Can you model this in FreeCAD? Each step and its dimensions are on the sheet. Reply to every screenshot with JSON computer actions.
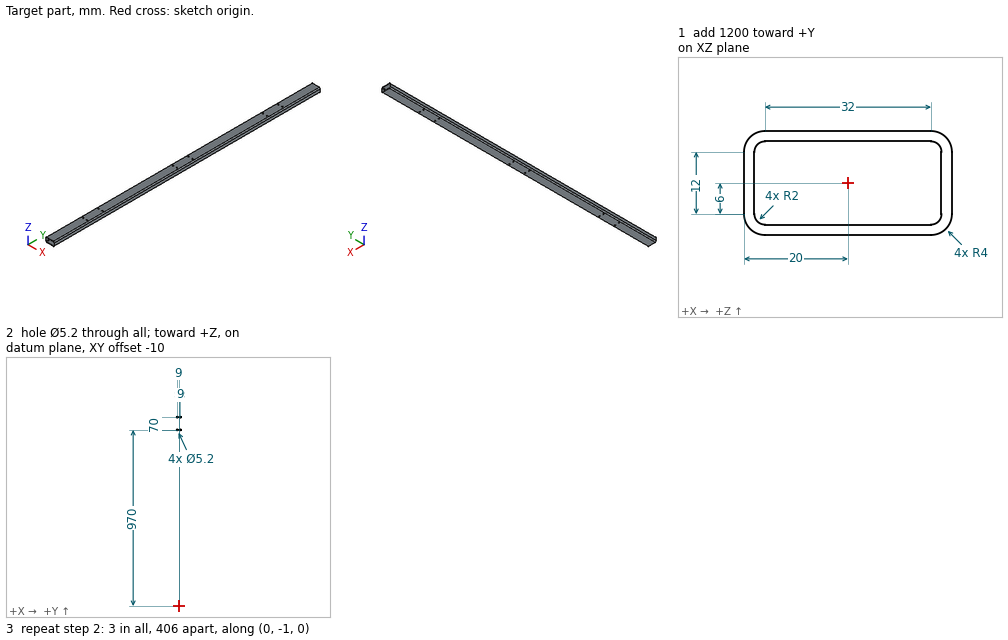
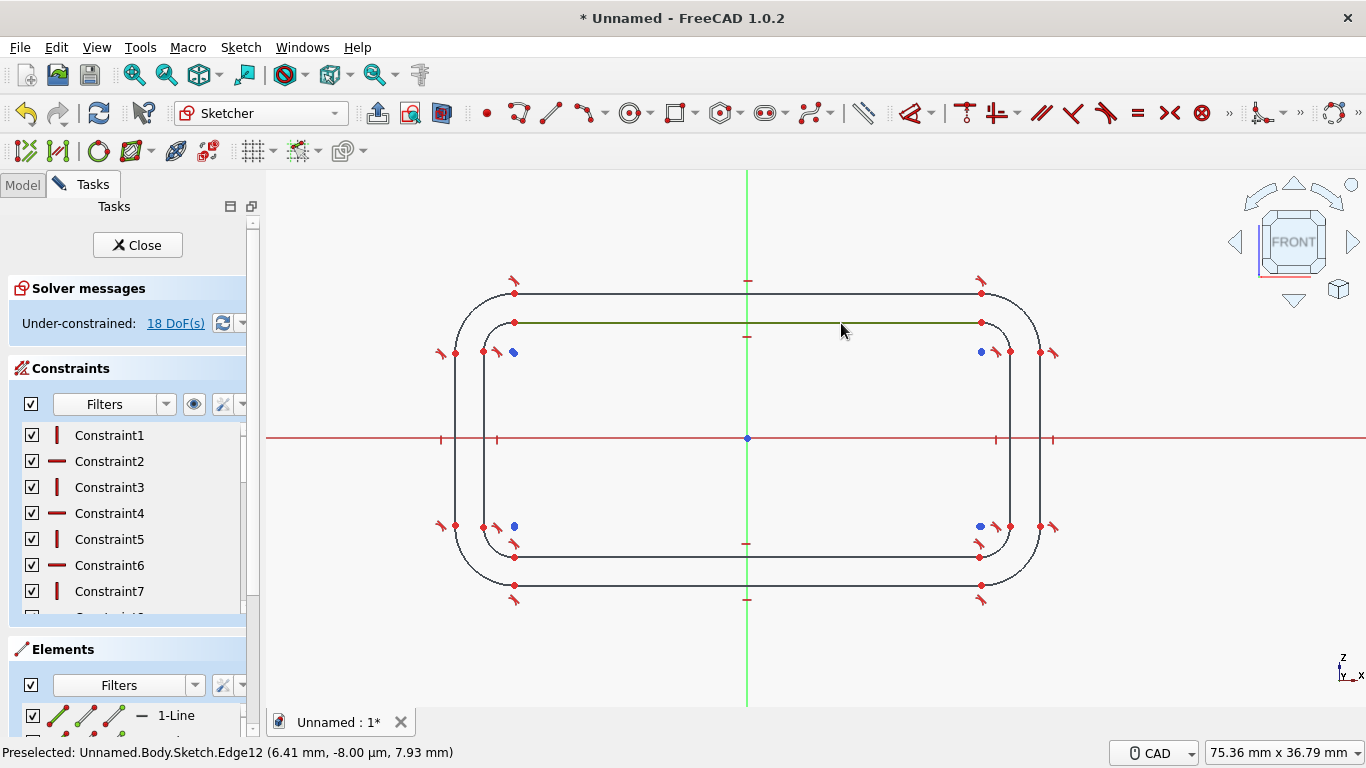
{"action": "left_click", "coordinate": [1007, 338]}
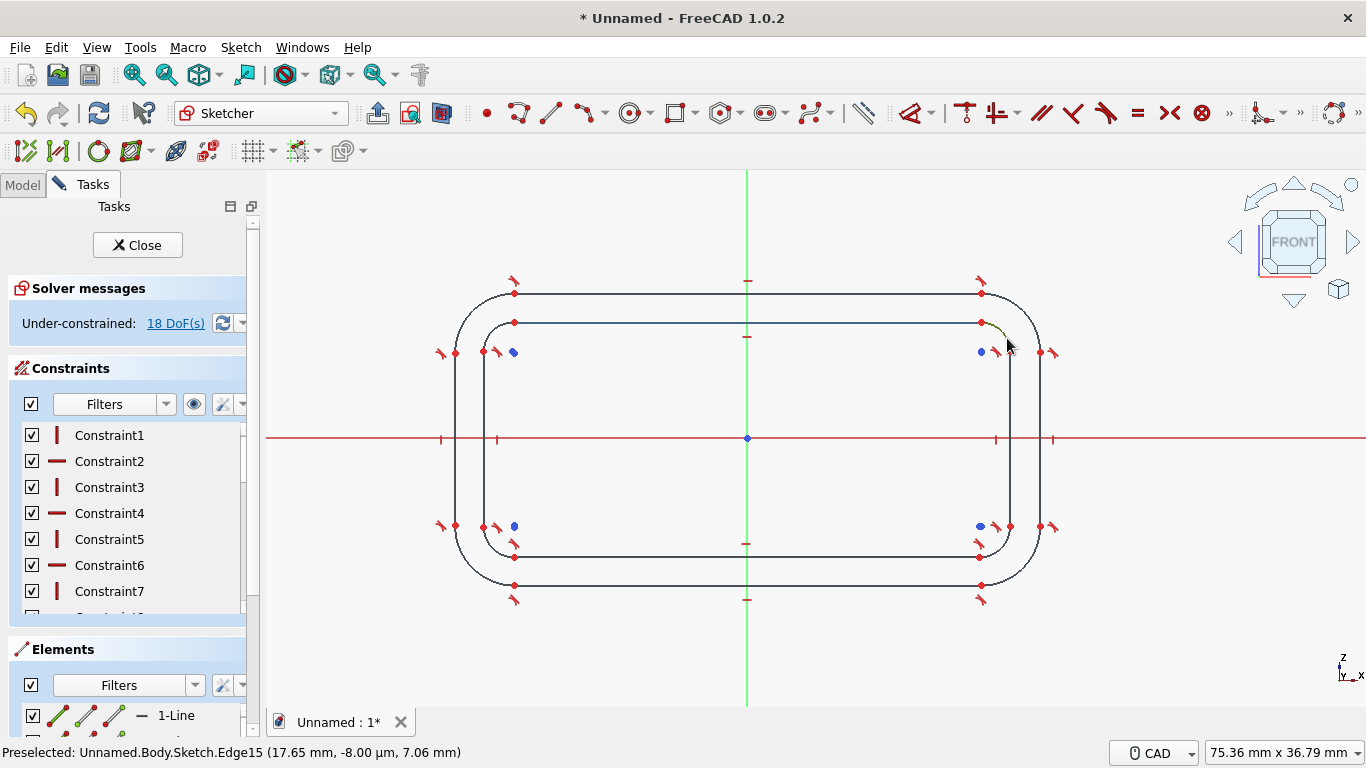
{"action": "left_click", "coordinate": [1106, 114]}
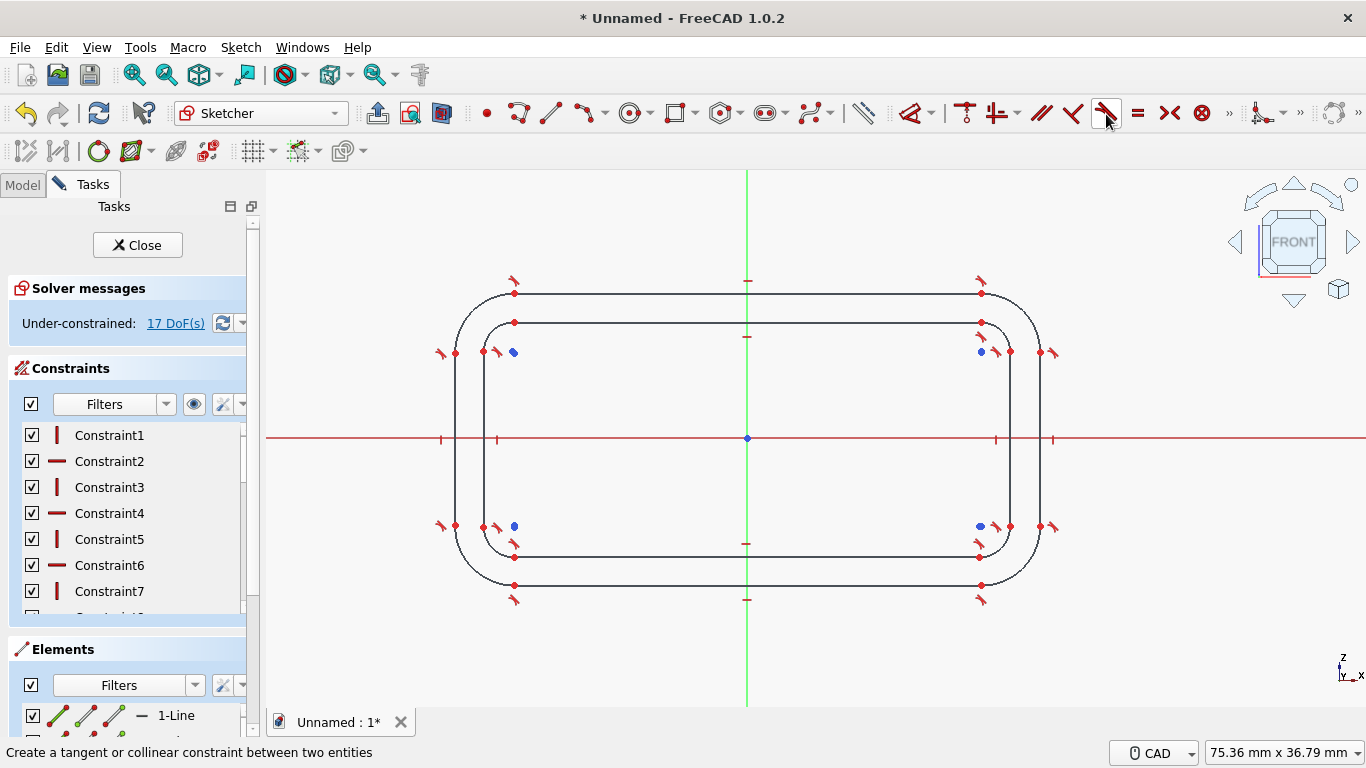
{"action": "left_click", "coordinate": [841, 323]}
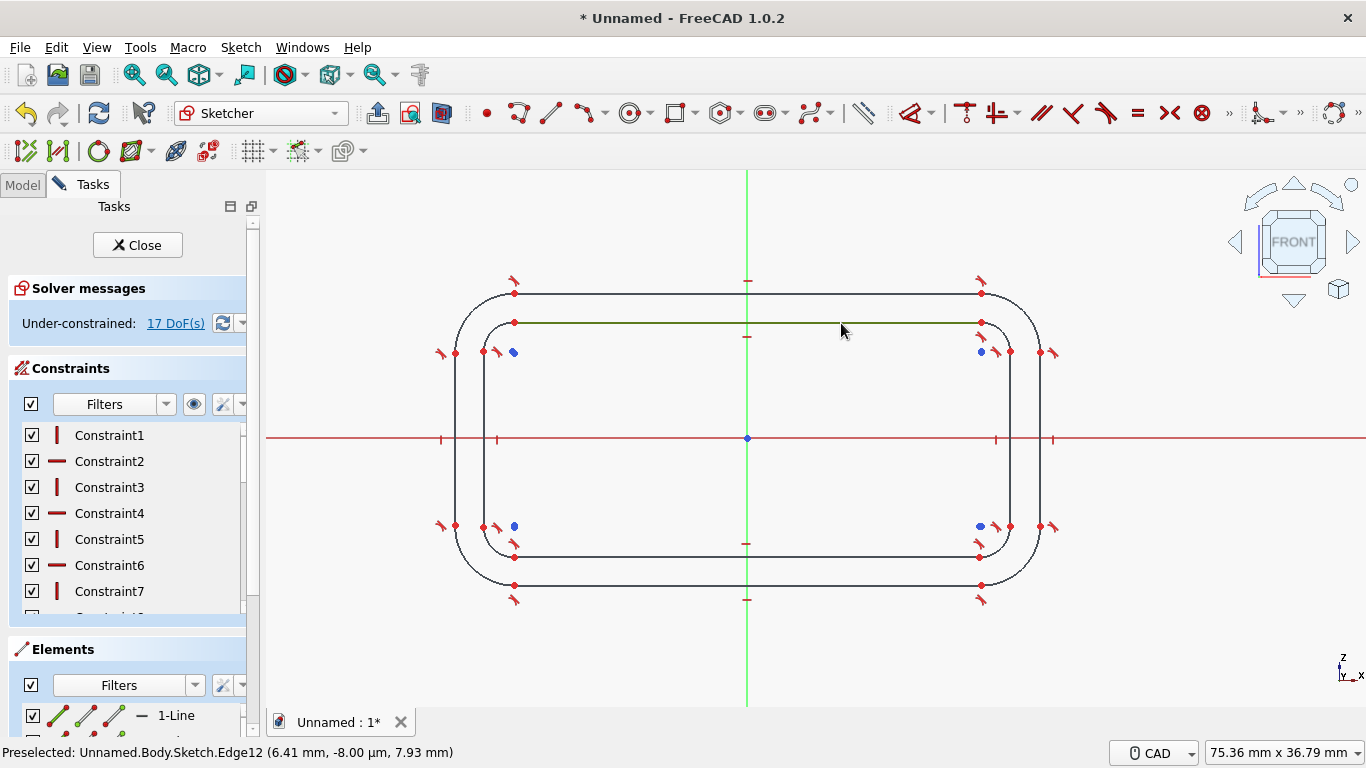
{"action": "left_click", "coordinate": [500, 325]}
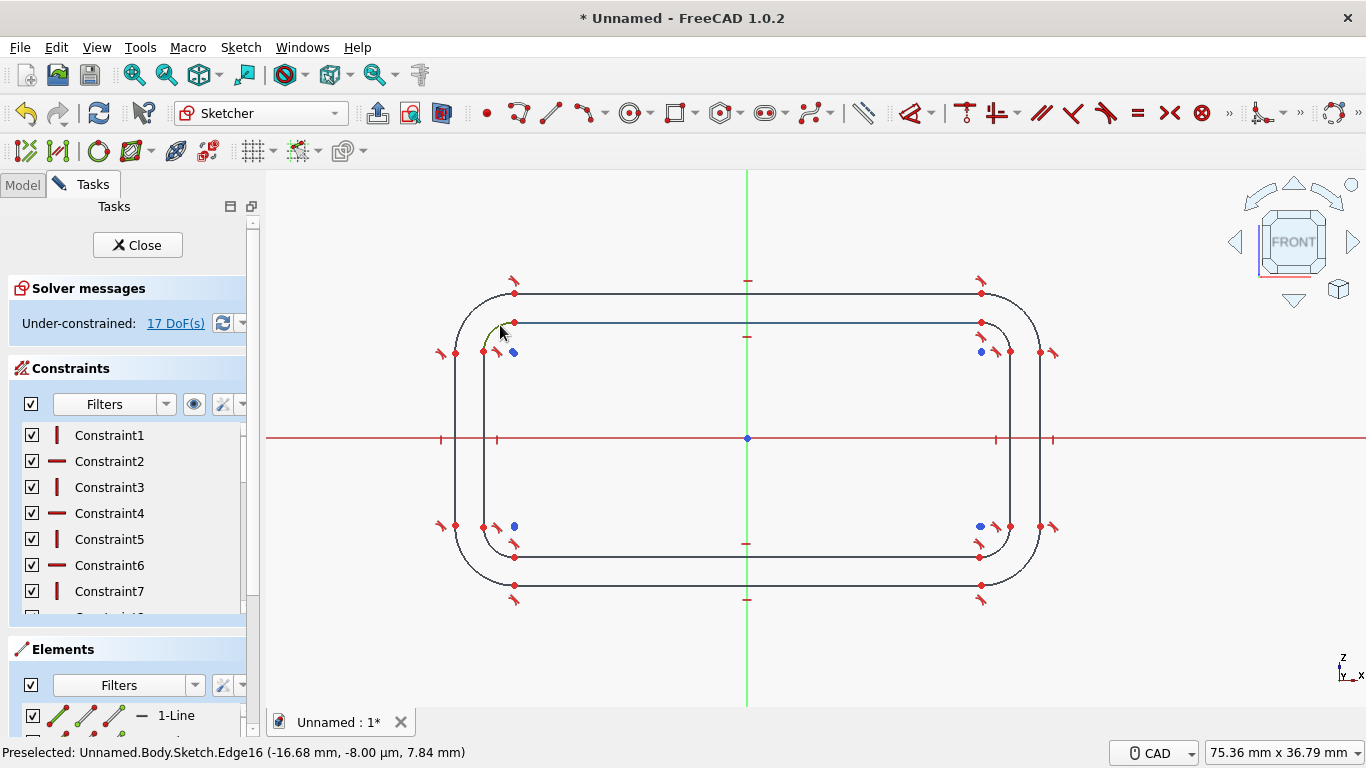
{"action": "left_click", "coordinate": [1106, 114]}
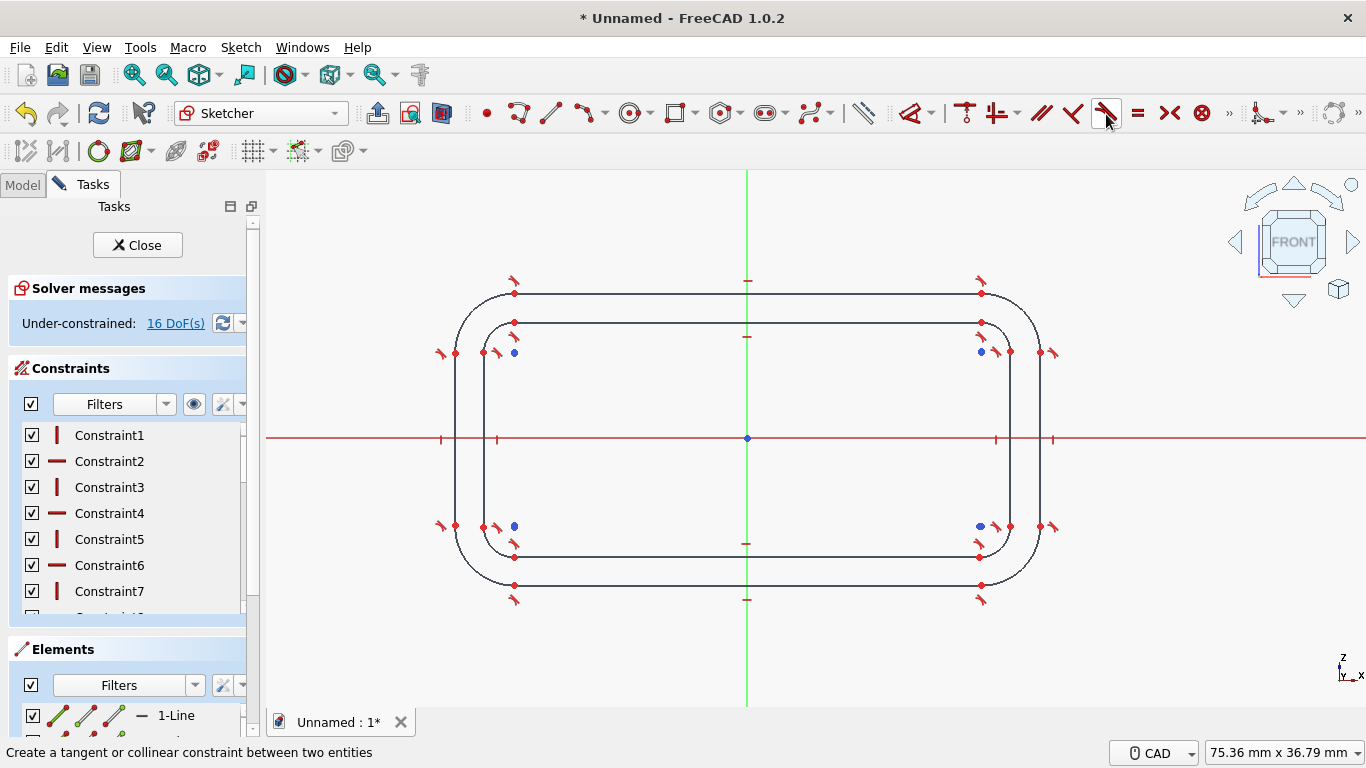
{"action": "left_click", "coordinate": [462, 553]}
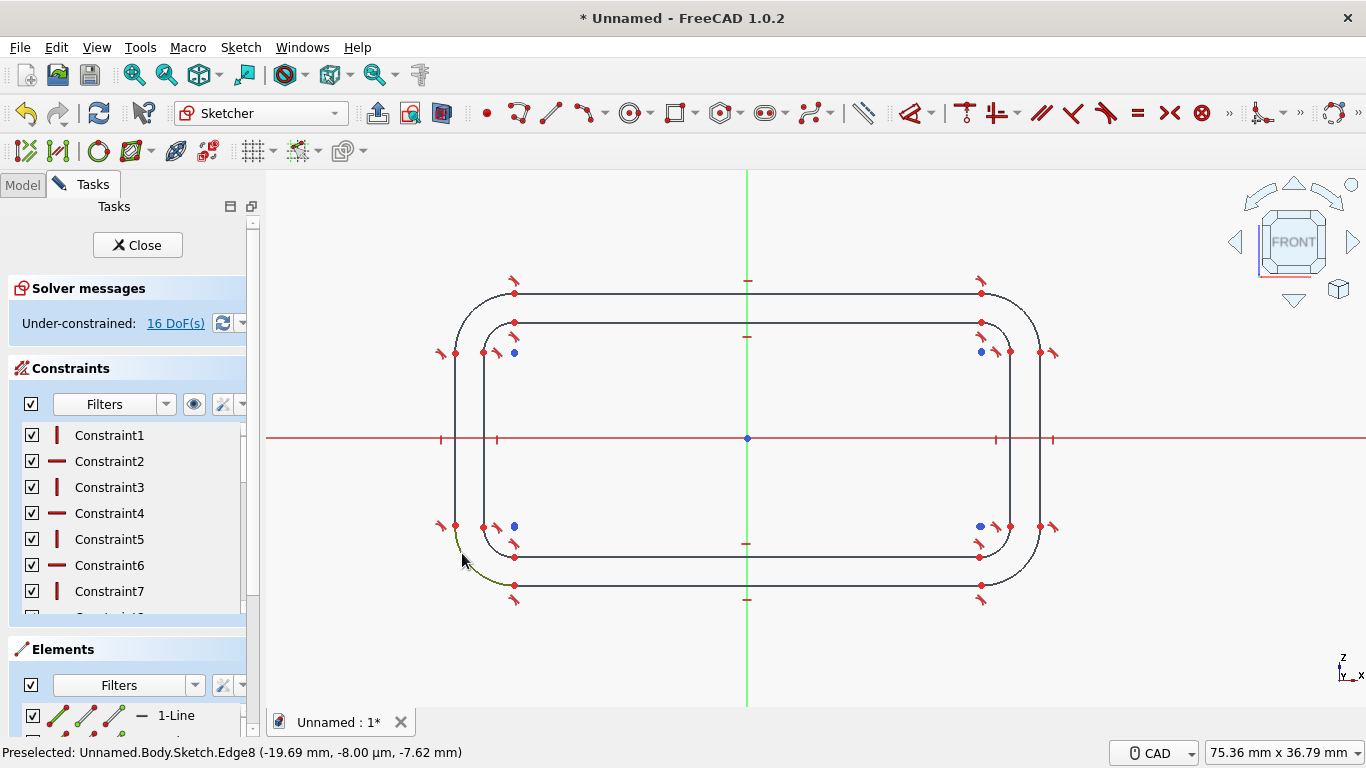
{"action": "left_click", "coordinate": [487, 541]}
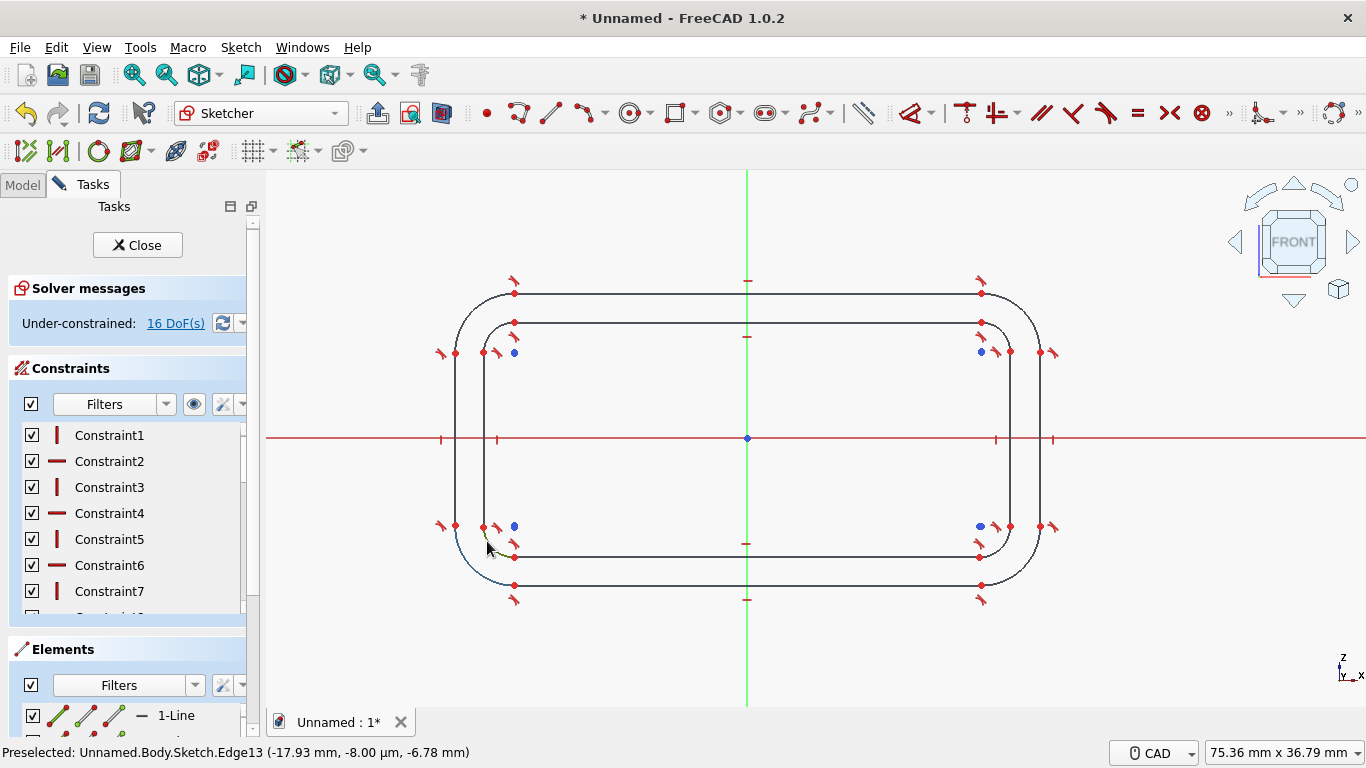
{"action": "left_click", "coordinate": [966, 114]}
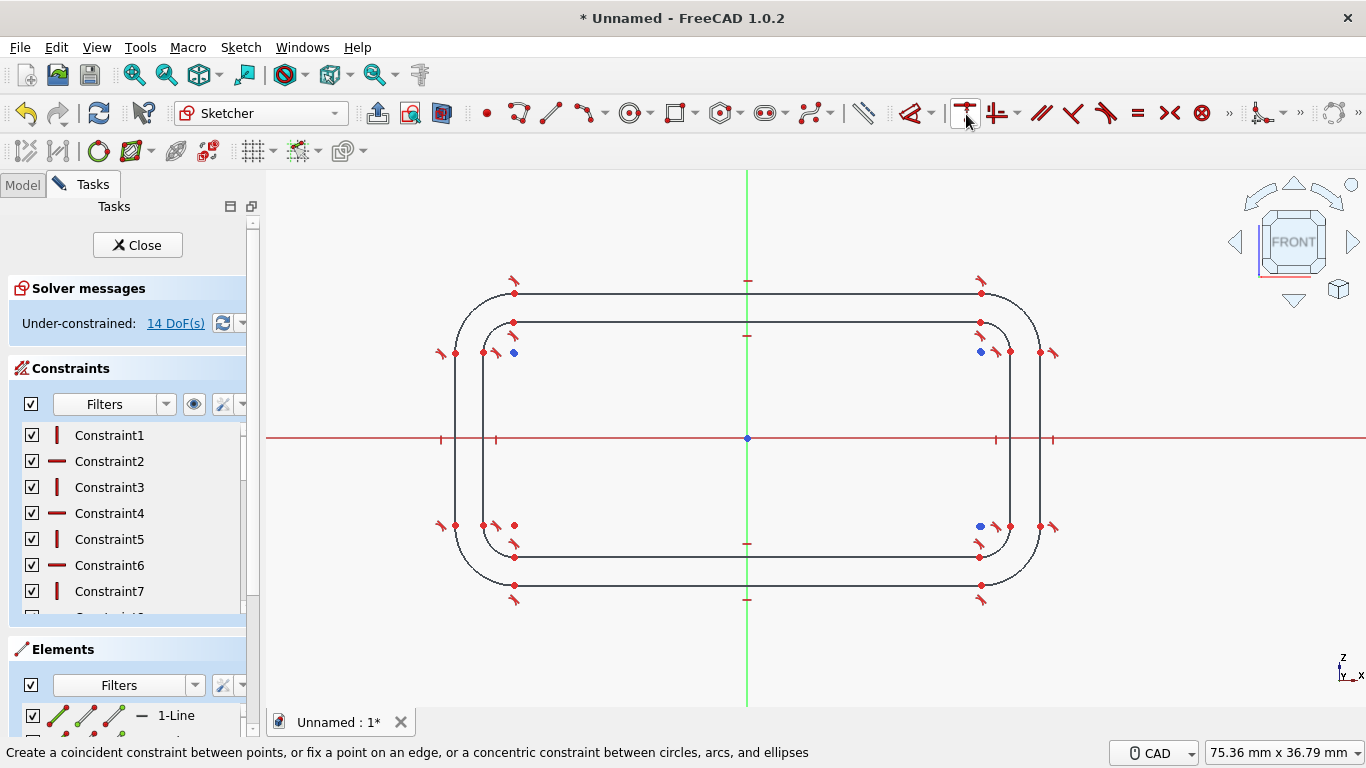
{"action": "left_click", "coordinate": [1008, 579]}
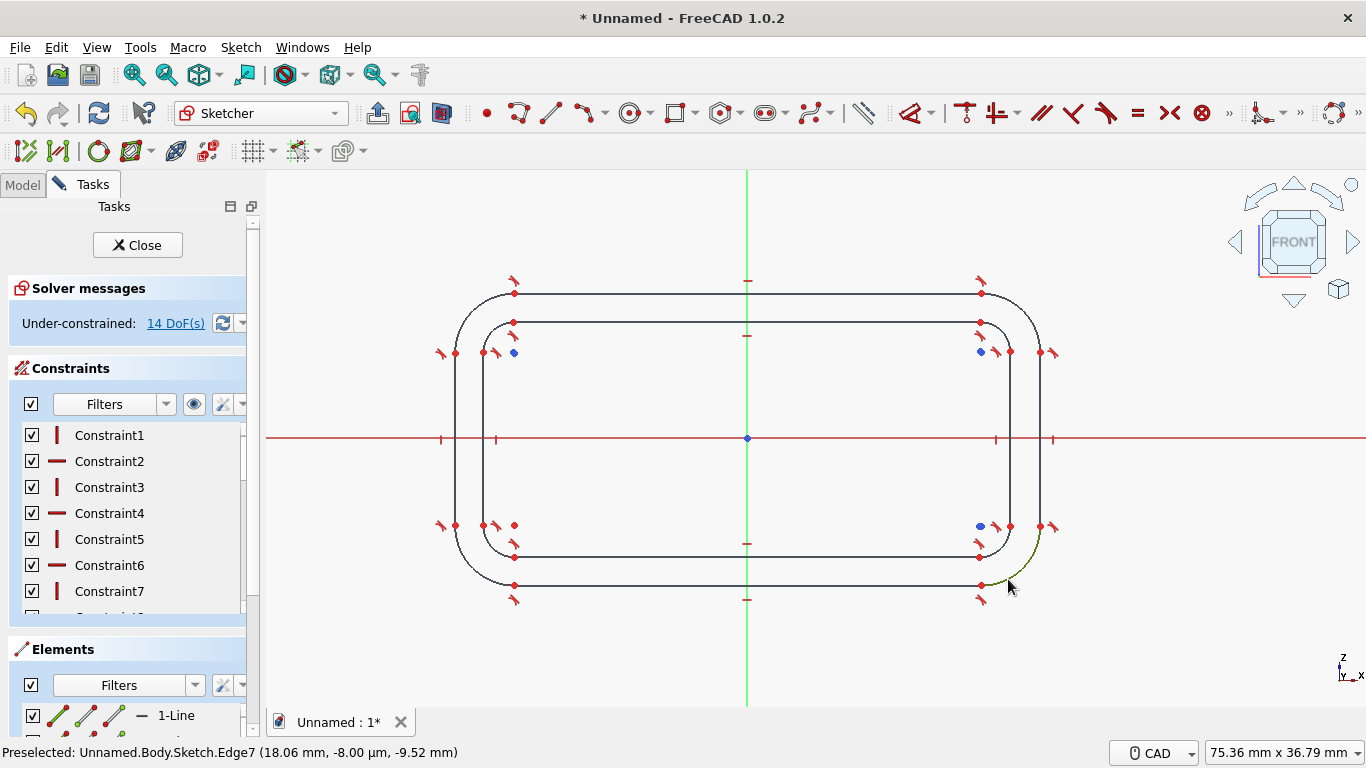
{"action": "left_click", "coordinate": [993, 554]}